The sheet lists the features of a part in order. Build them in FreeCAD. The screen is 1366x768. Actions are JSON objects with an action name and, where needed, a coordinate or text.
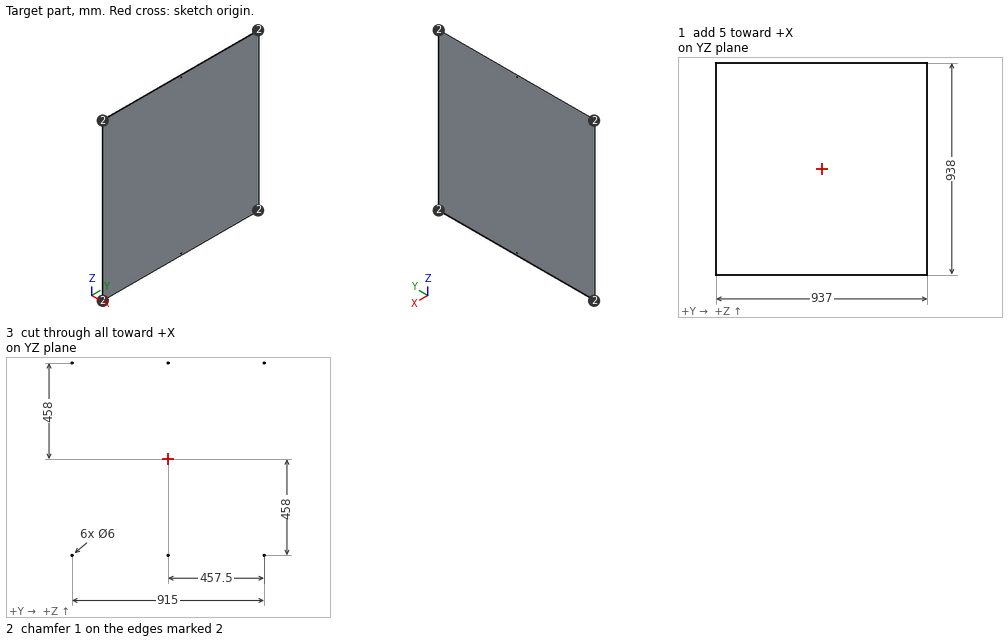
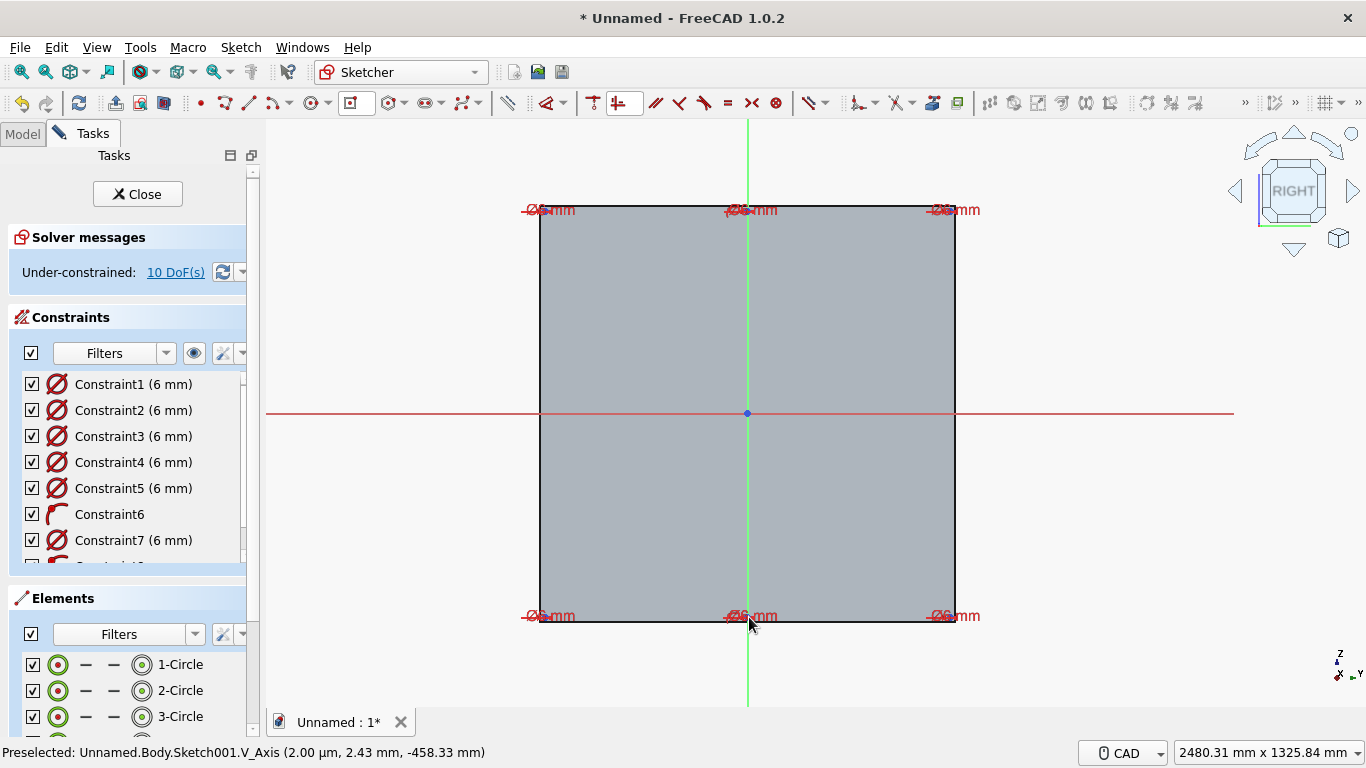
{"action": "left_click", "coordinate": [950, 618]}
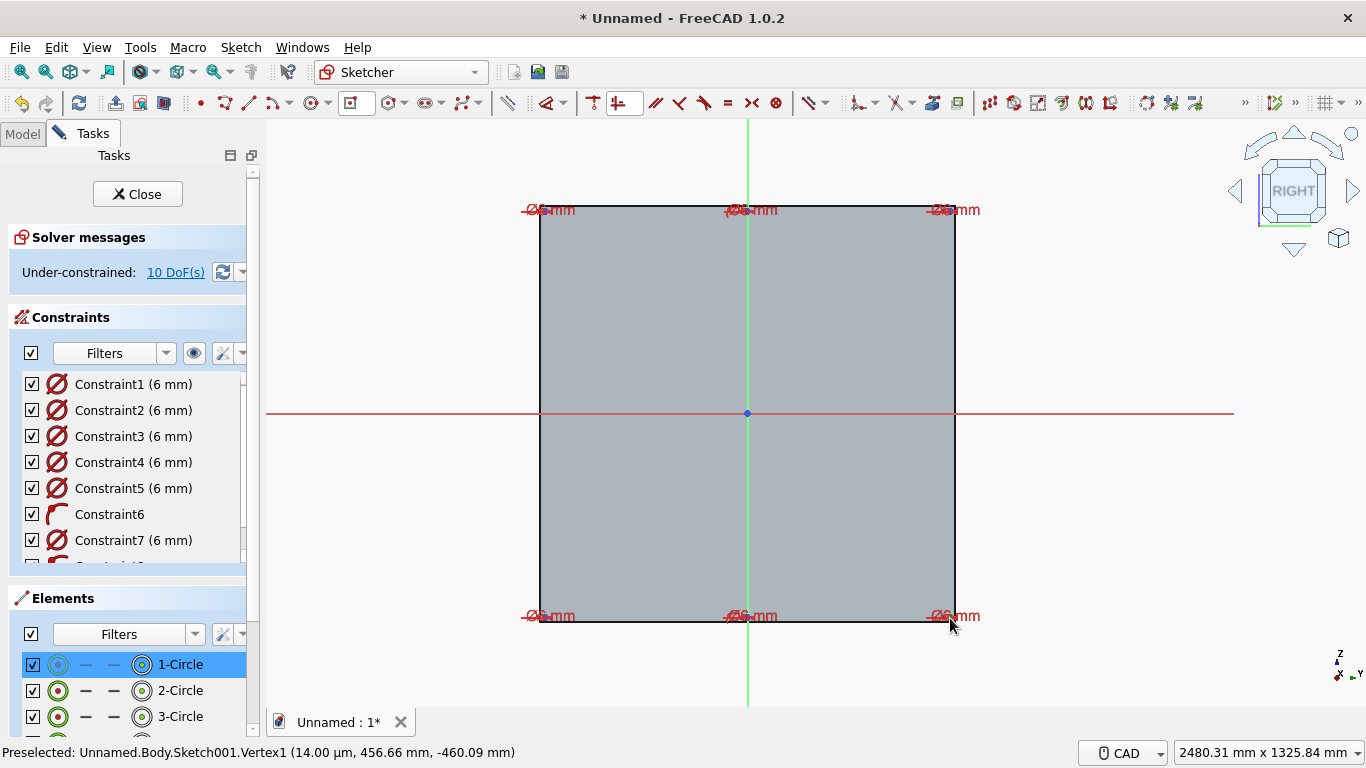
{"action": "left_click", "coordinate": [545, 618]}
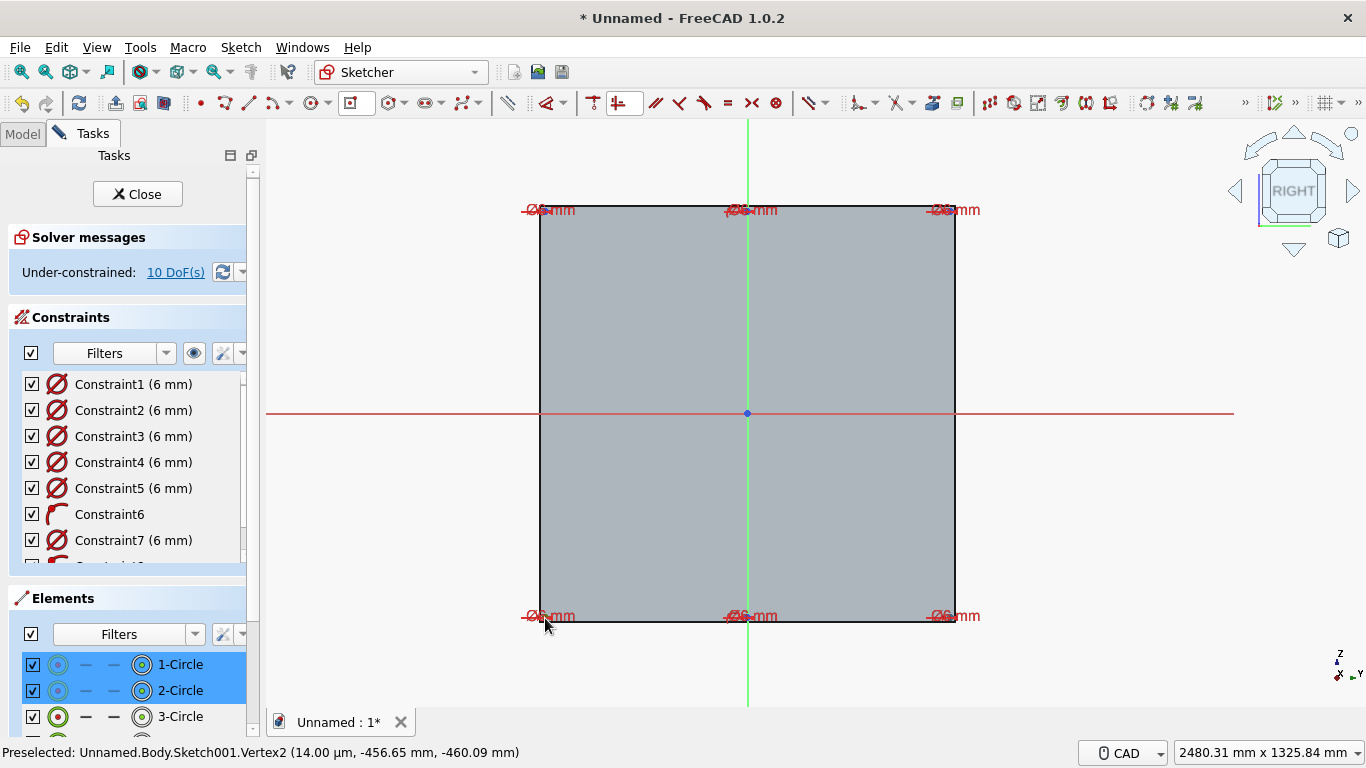
{"action": "left_click", "coordinate": [638, 104]}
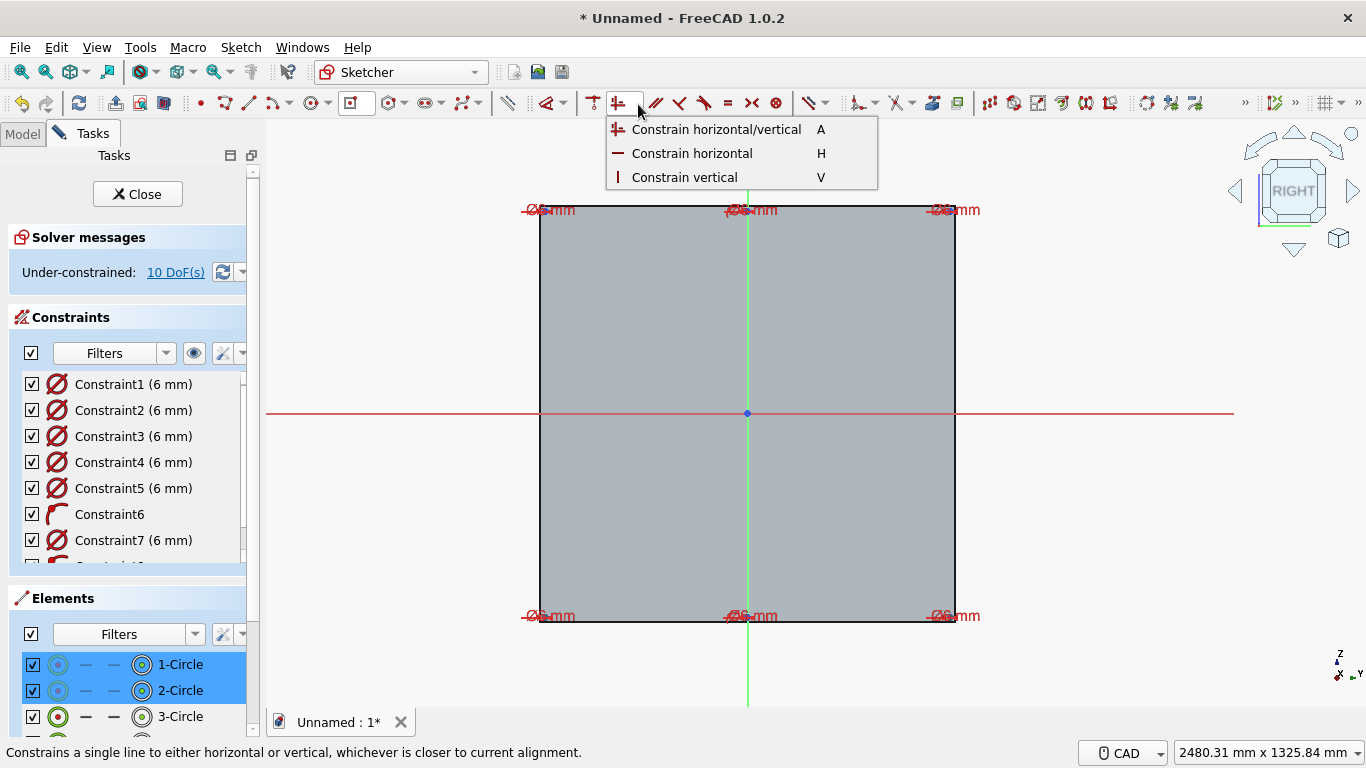
{"action": "left_click", "coordinate": [742, 153]}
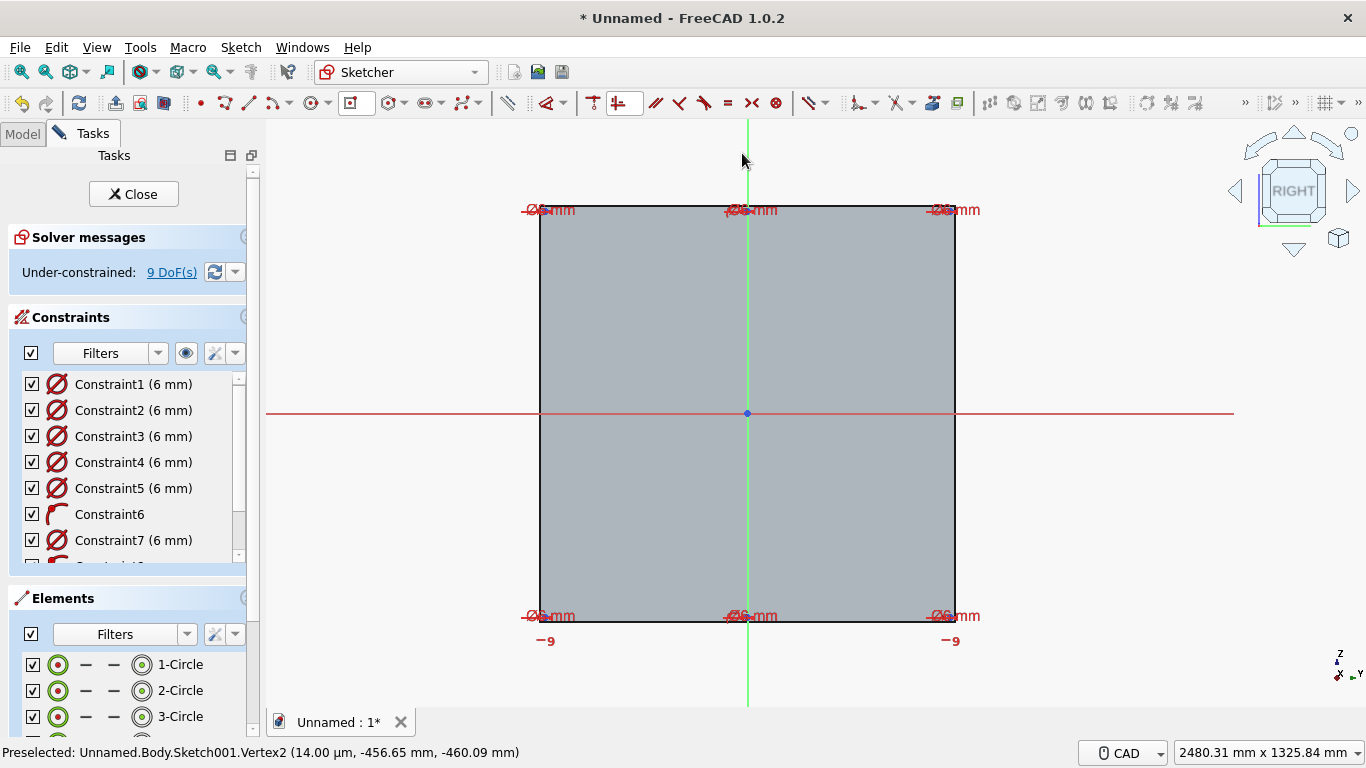
{"action": "left_click", "coordinate": [545, 618]}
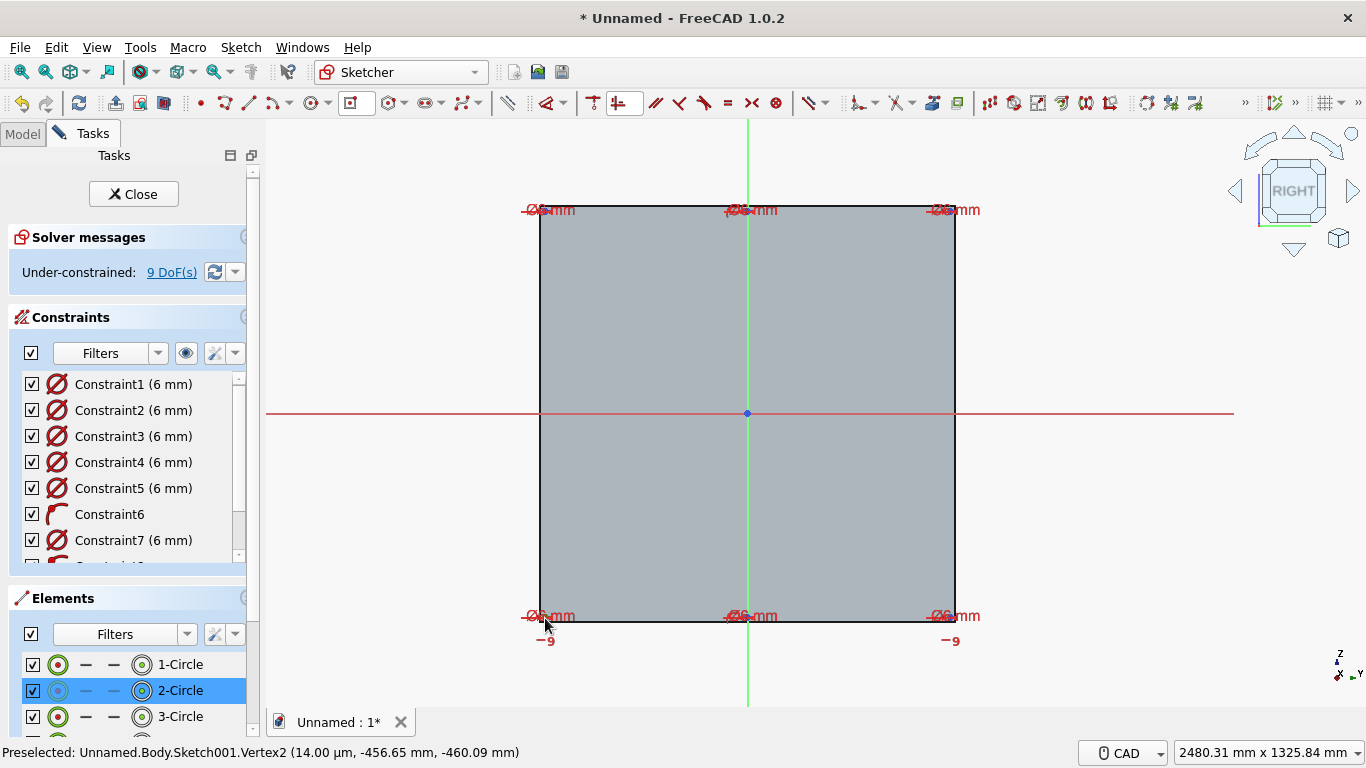
{"action": "left_click", "coordinate": [545, 212]}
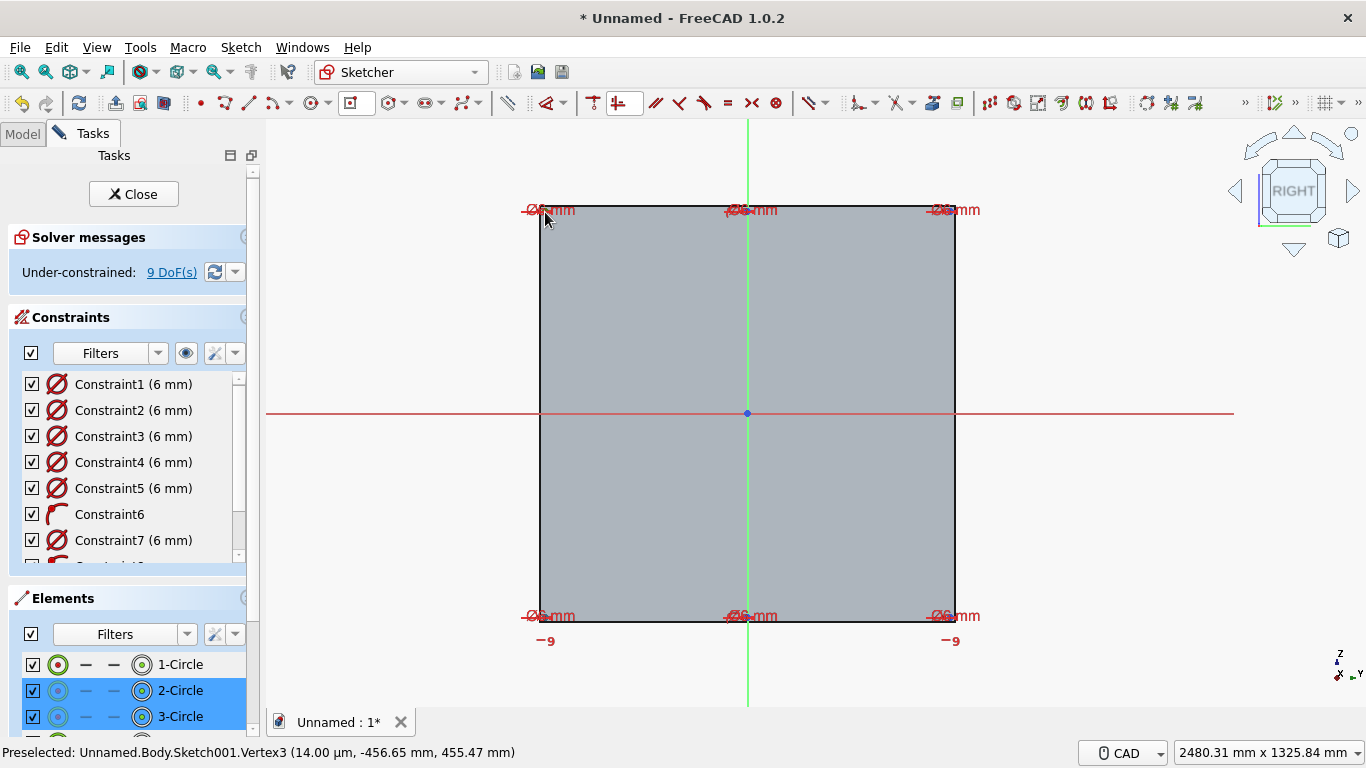
{"action": "left_click", "coordinate": [638, 104]}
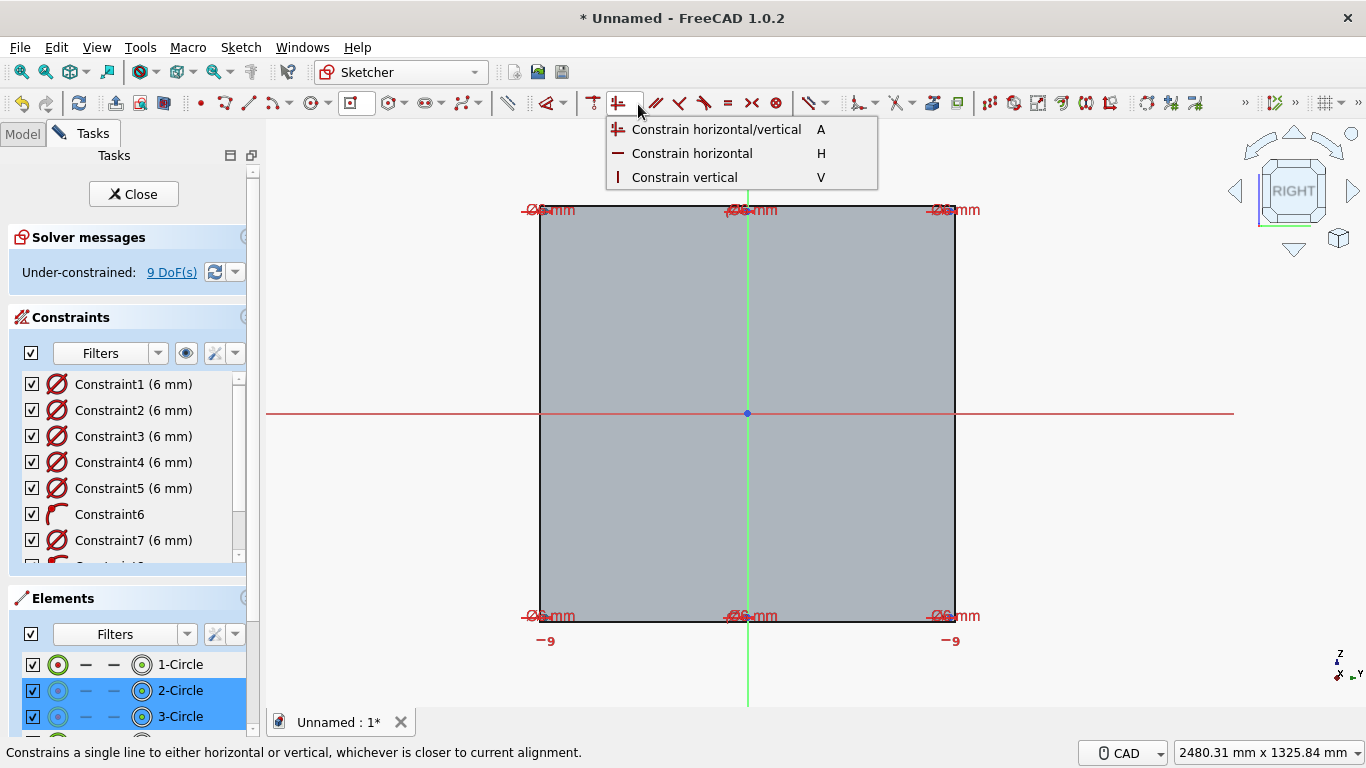
{"action": "left_click", "coordinate": [742, 177]}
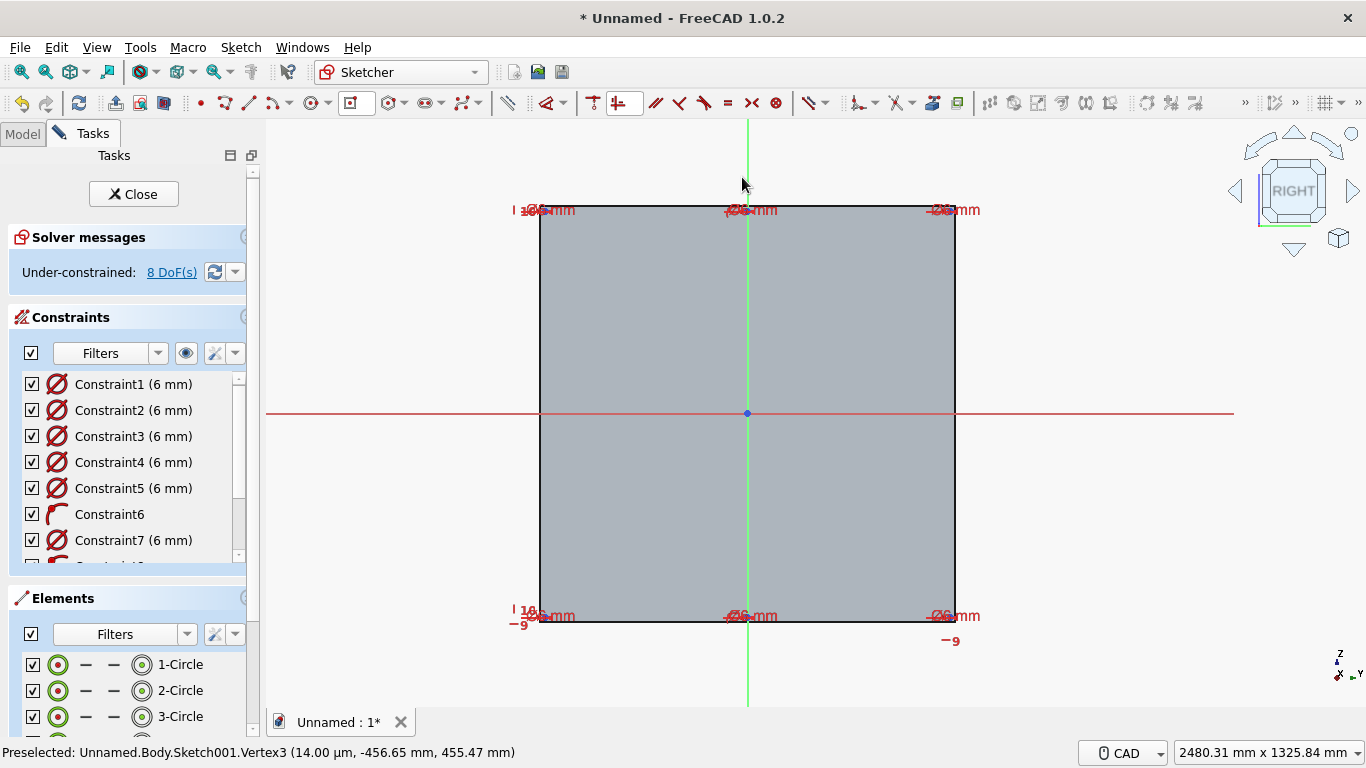
{"action": "left_click", "coordinate": [950, 618]}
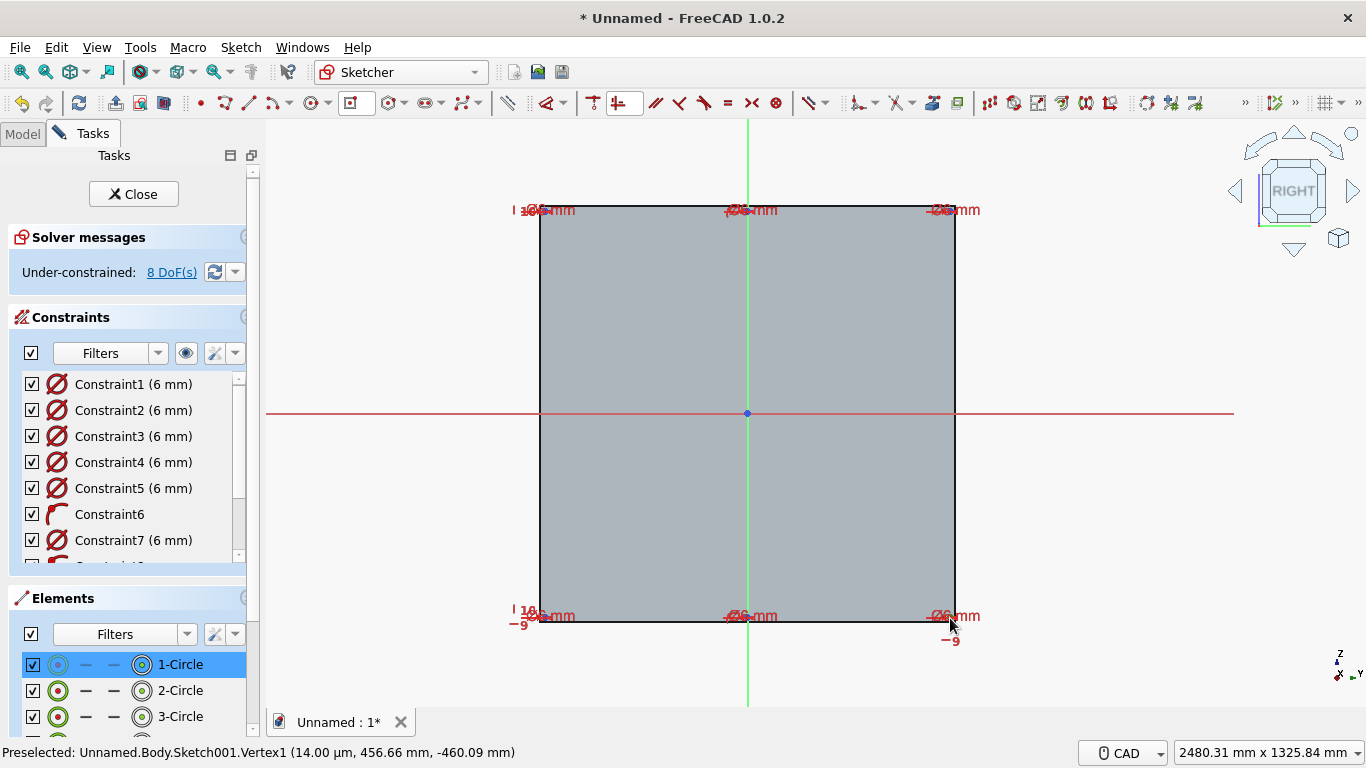
{"action": "left_click", "coordinate": [950, 212]}